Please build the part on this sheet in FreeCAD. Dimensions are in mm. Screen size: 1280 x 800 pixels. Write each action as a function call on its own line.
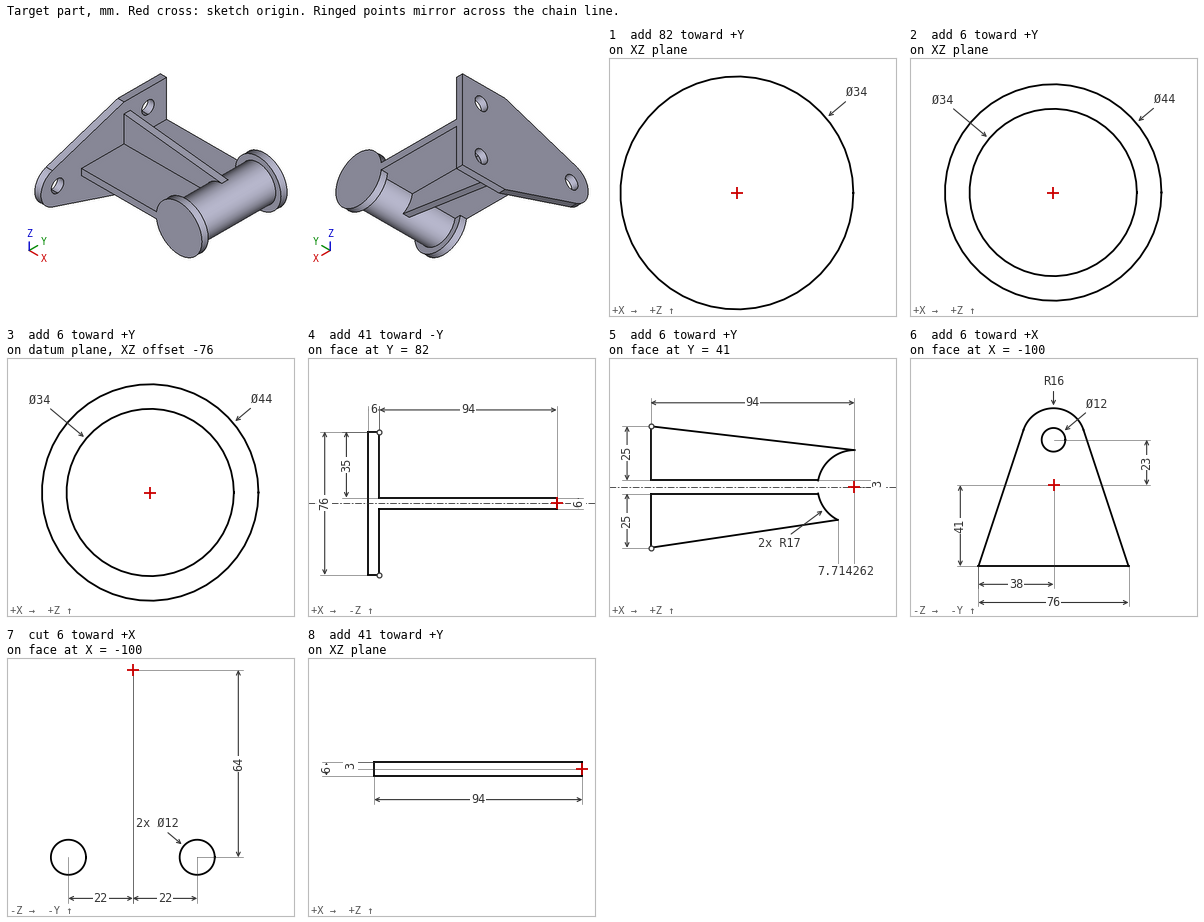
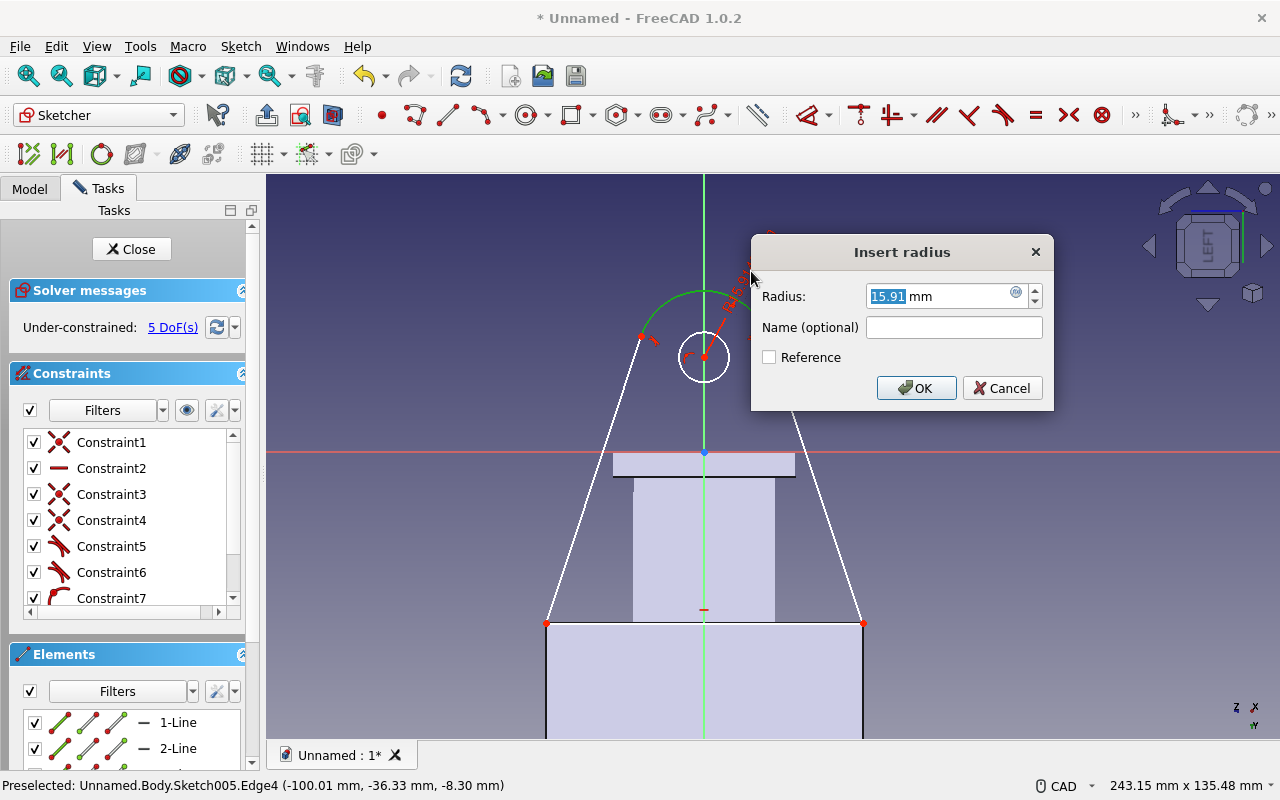
text(16)
key(Return)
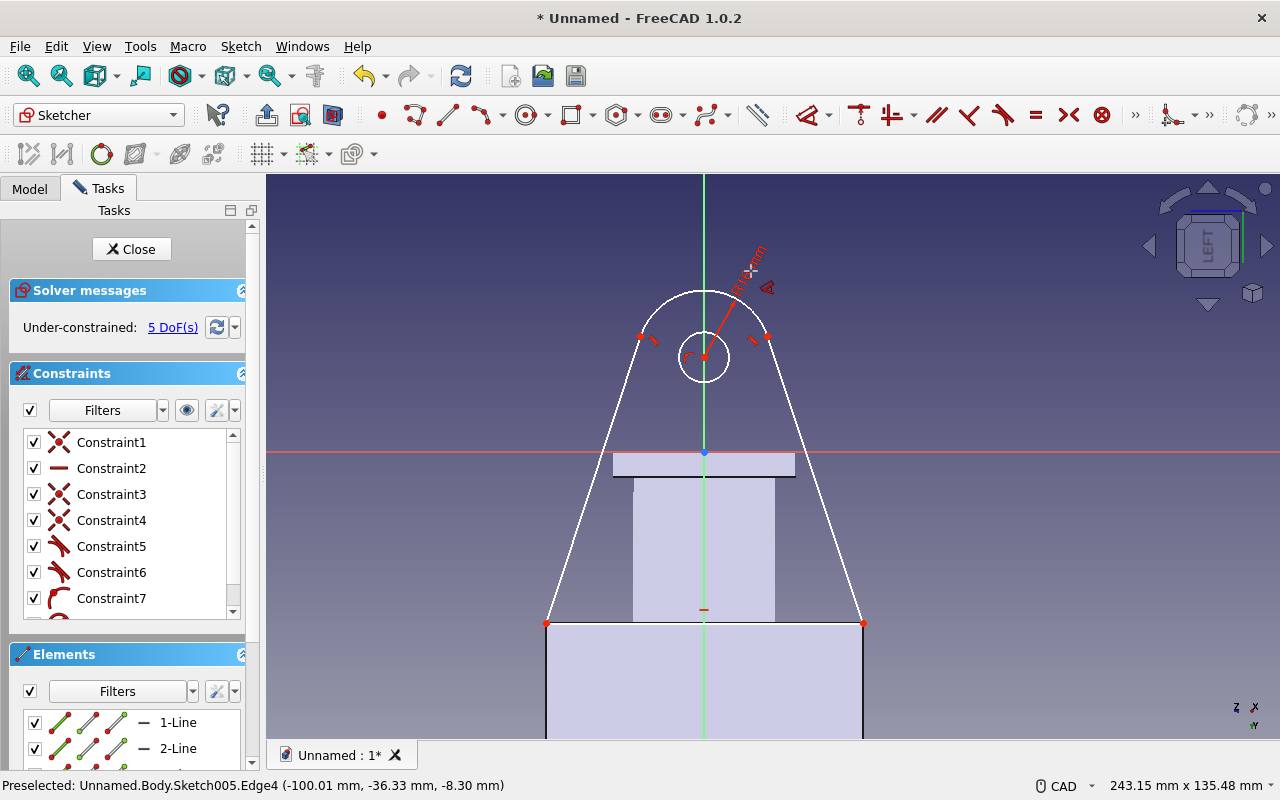
click(722, 340)
click(759, 370)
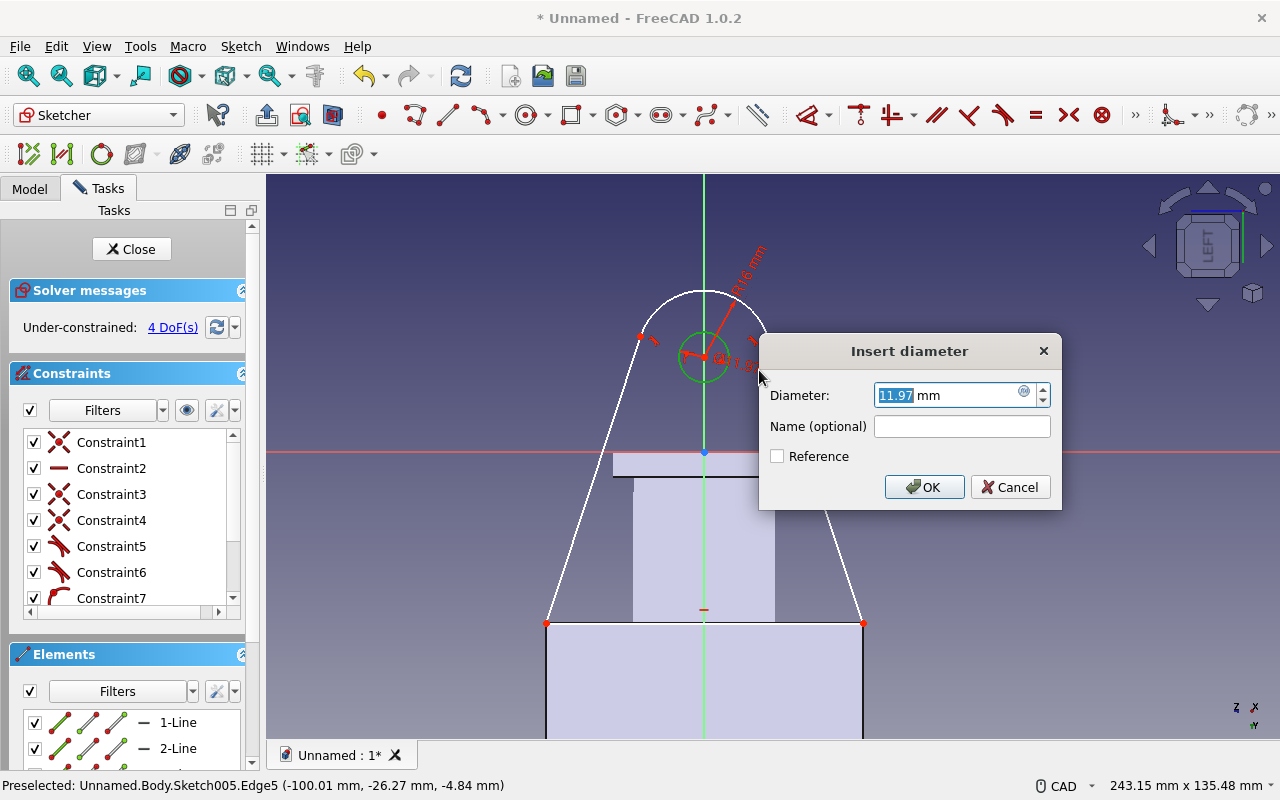
text(12)
key(Return)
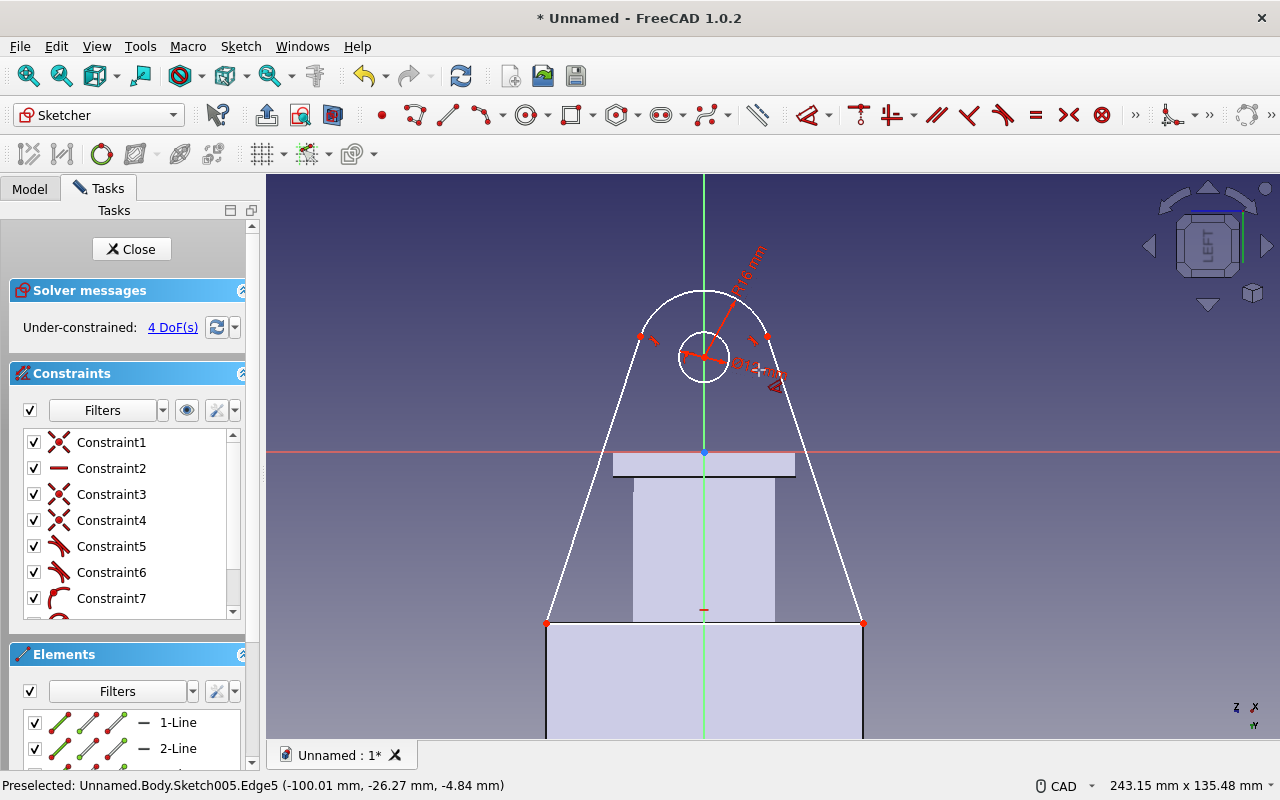
click(641, 624)
click(632, 658)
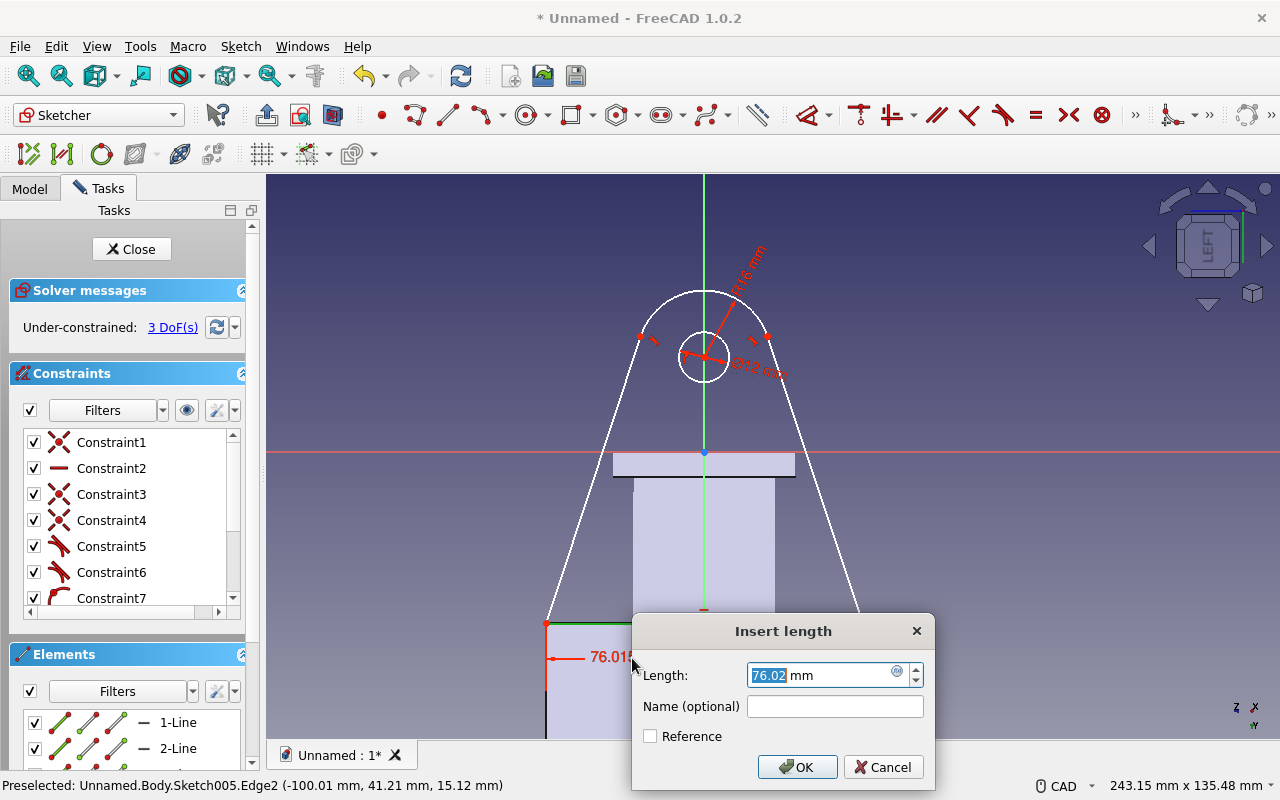
text(76)
key(Return)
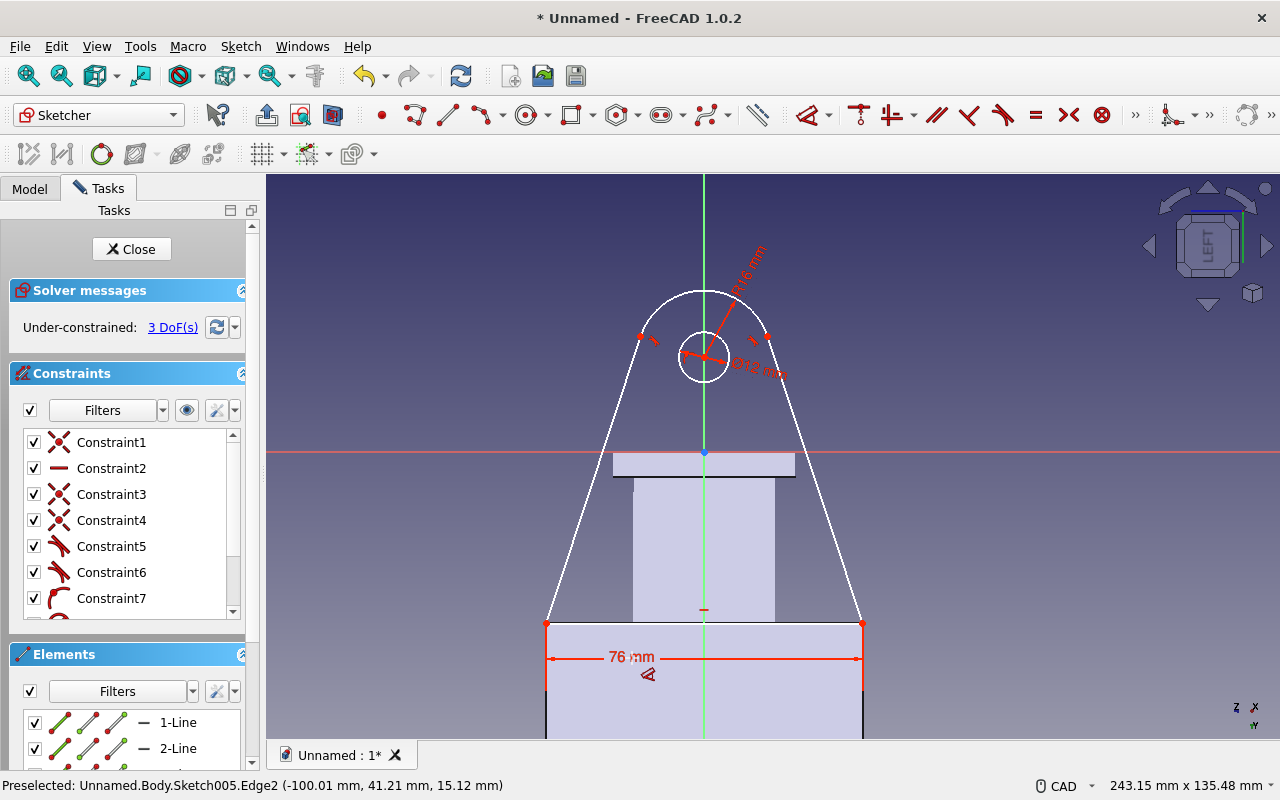
click(704, 357)
click(738, 405)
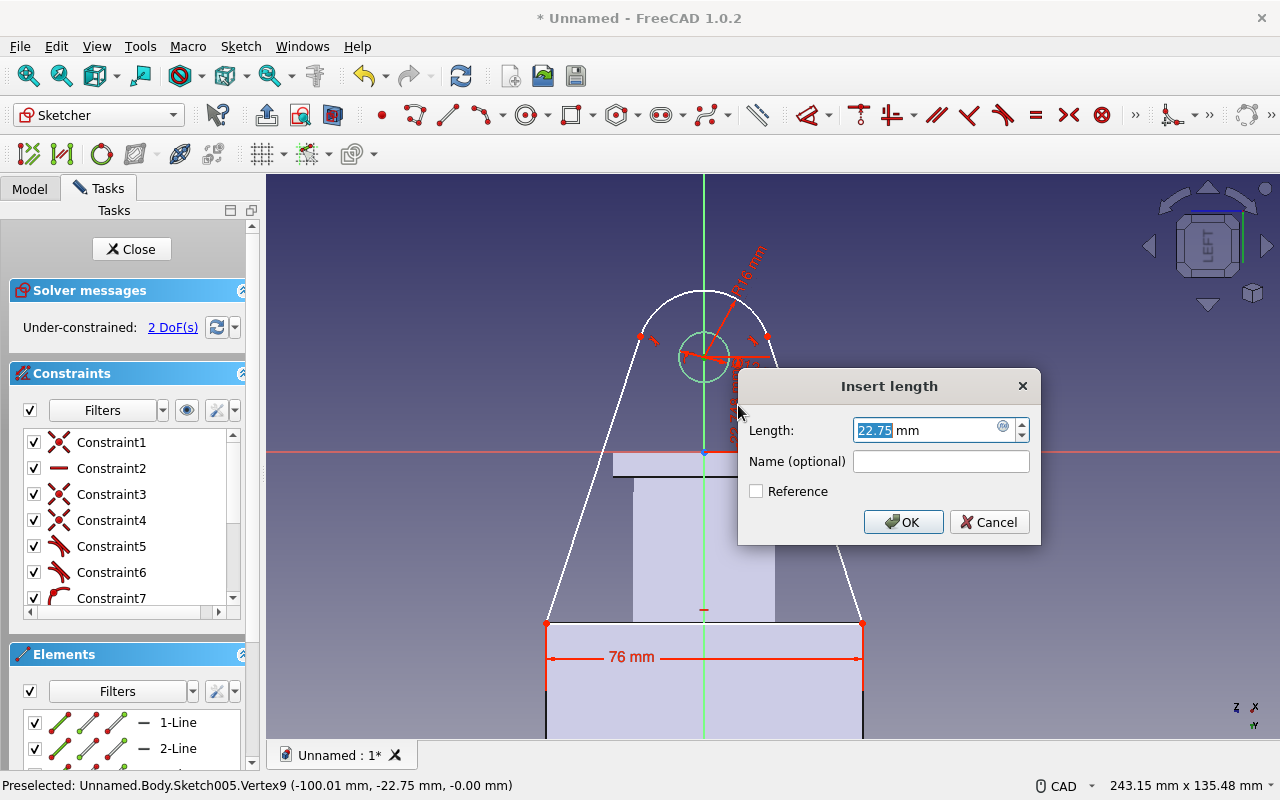
text(23)
key(Return)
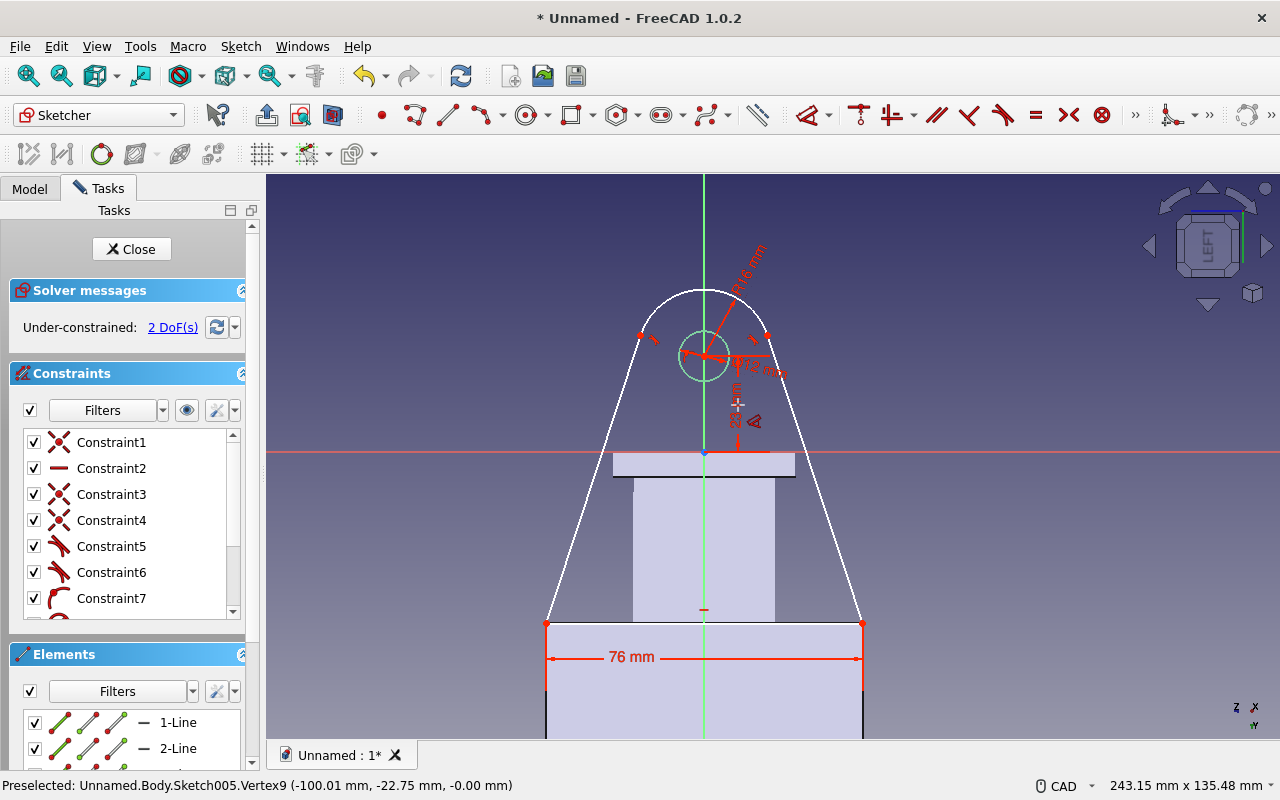
click(546, 624)
click(589, 418)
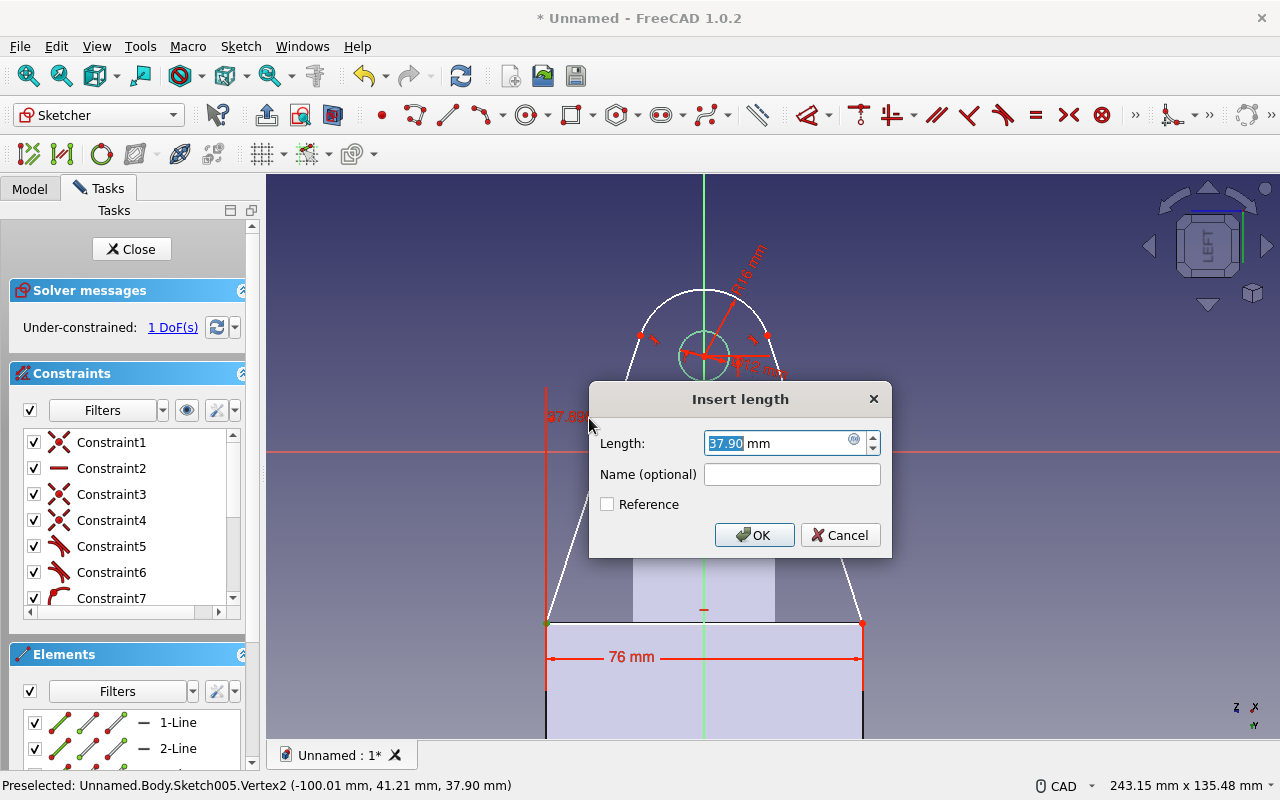
text(38)
key(Return)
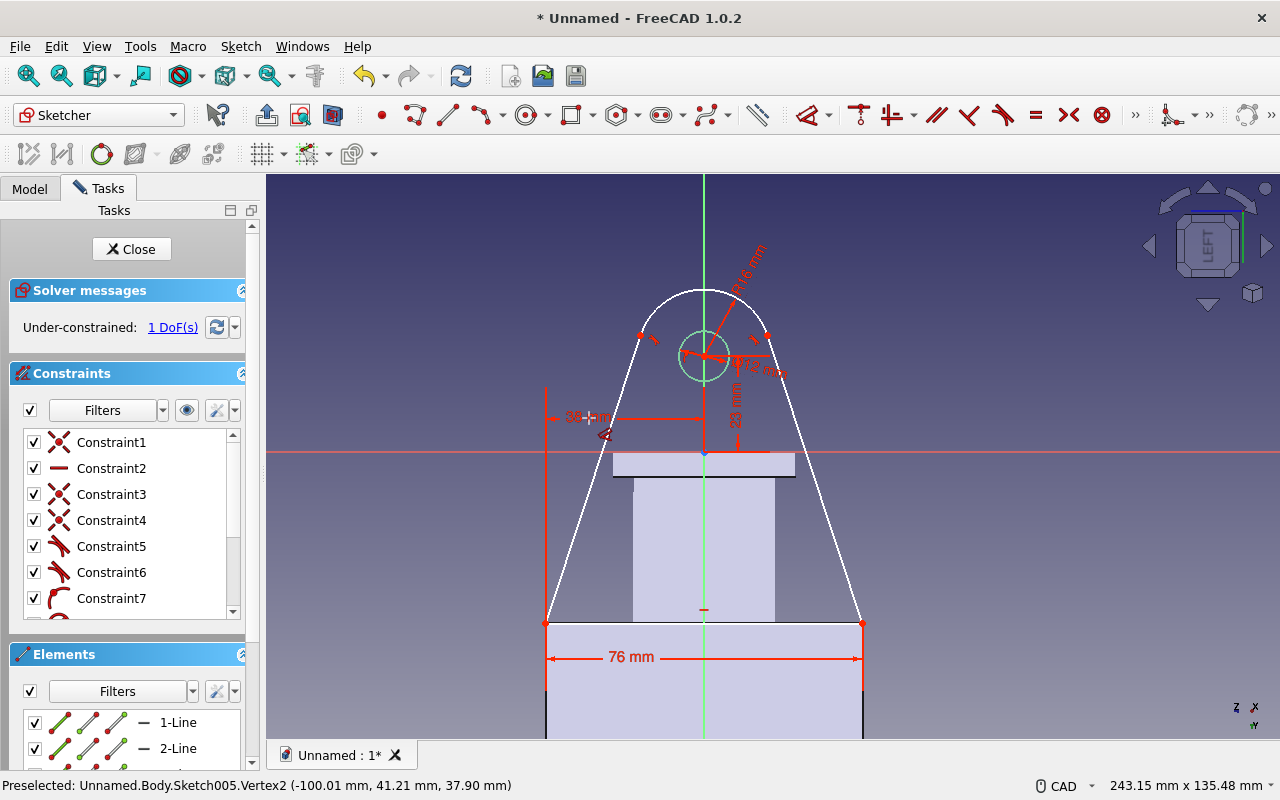
click(546, 624)
click(512, 538)